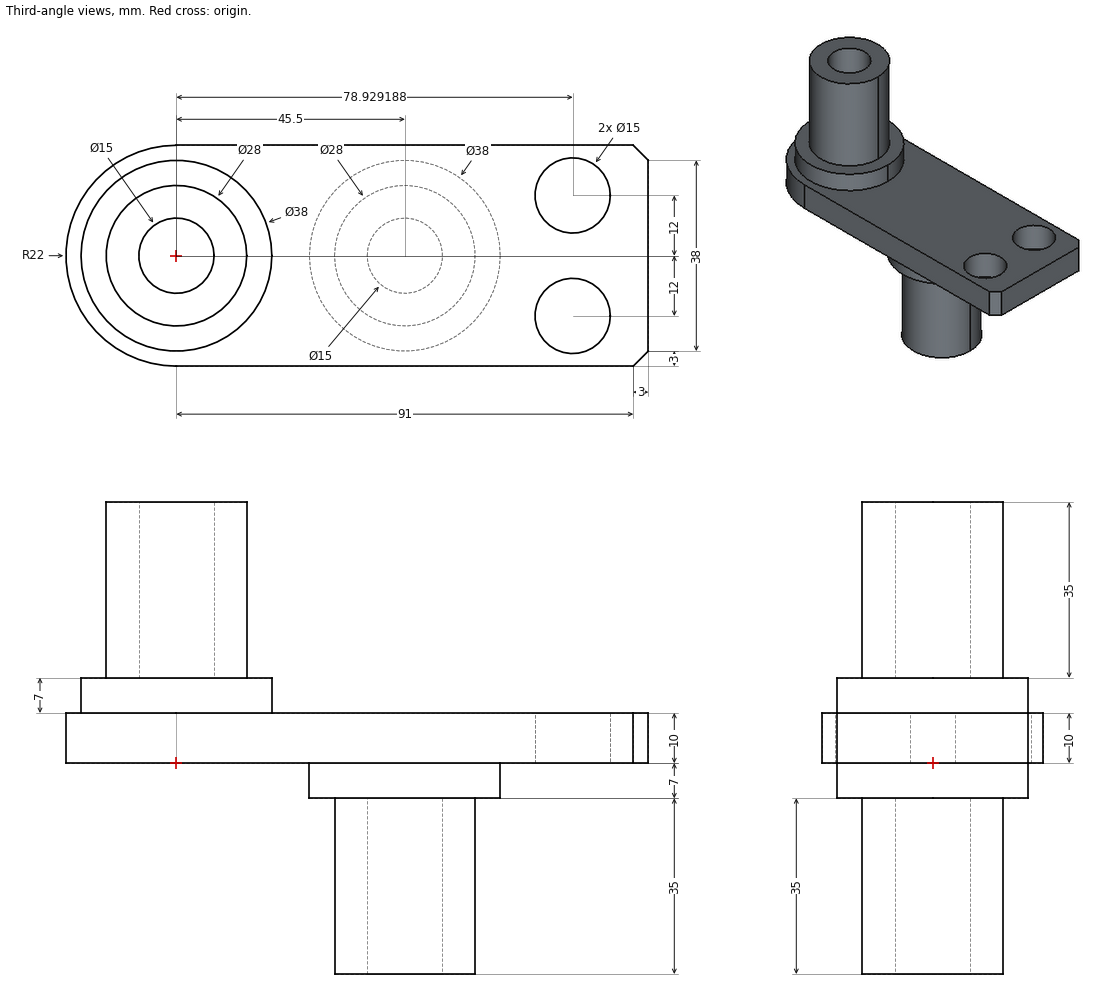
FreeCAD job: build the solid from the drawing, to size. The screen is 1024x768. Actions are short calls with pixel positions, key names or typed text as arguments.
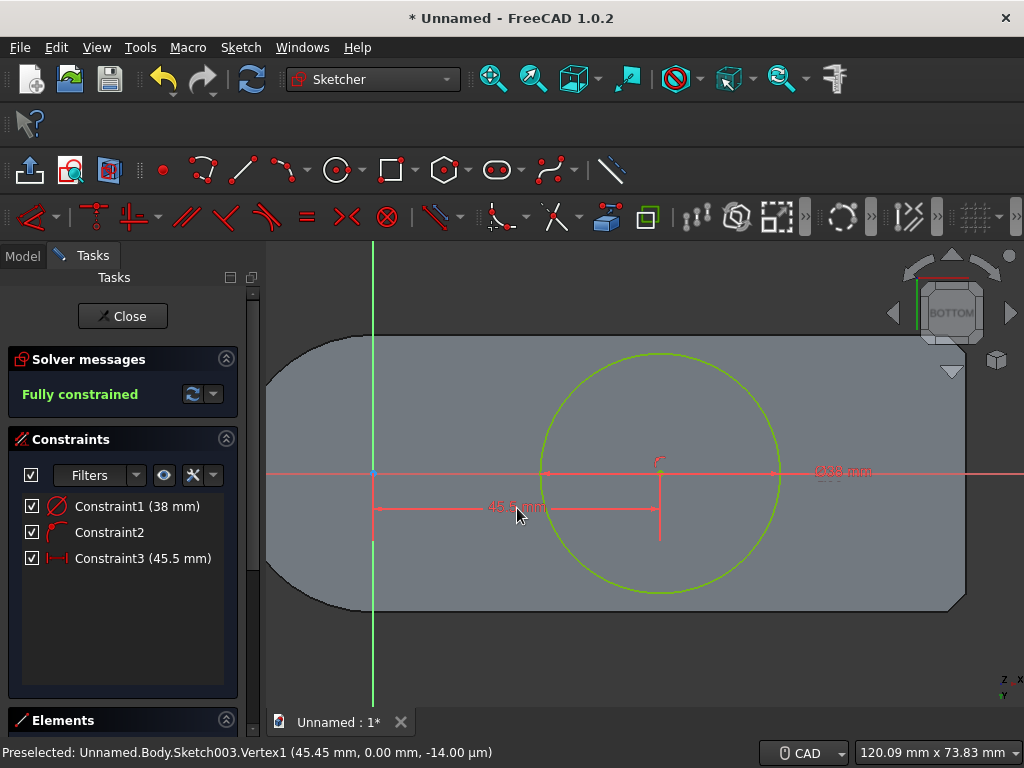
click(123, 316)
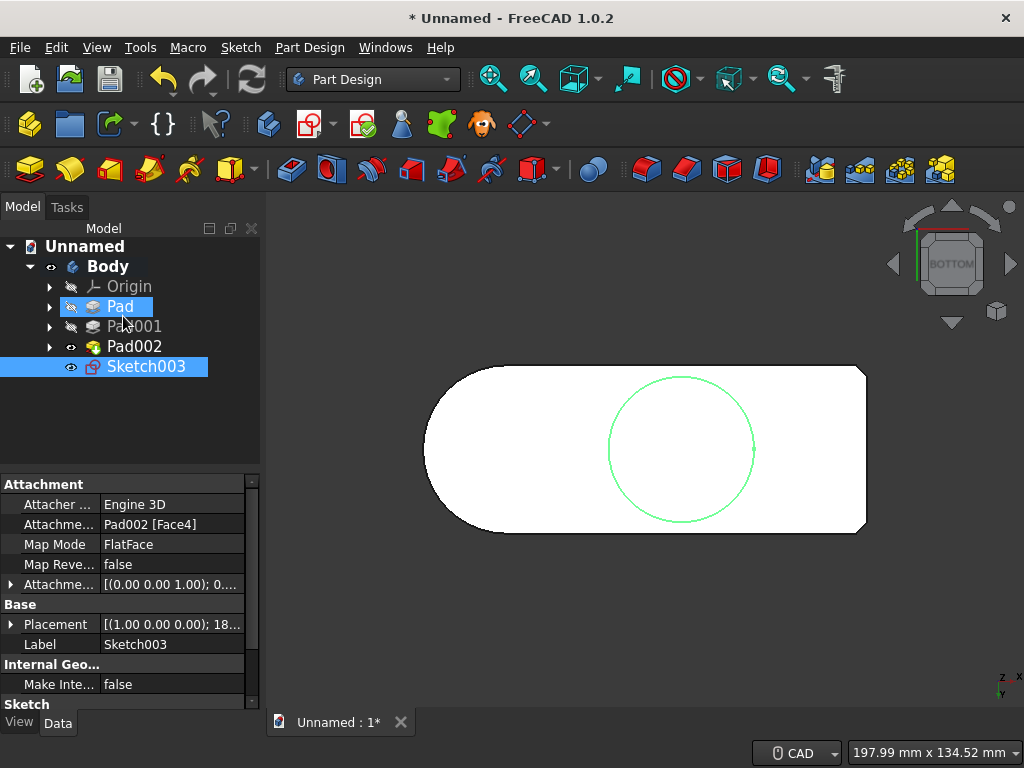
click(30, 170)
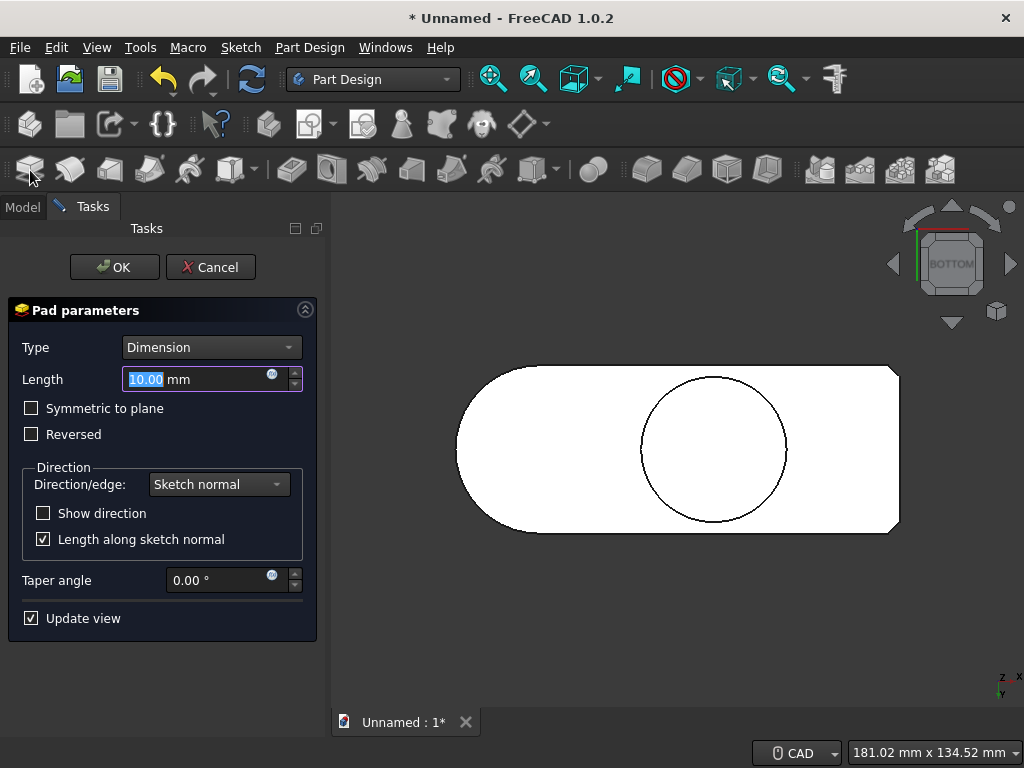
text(7)
key(Tab)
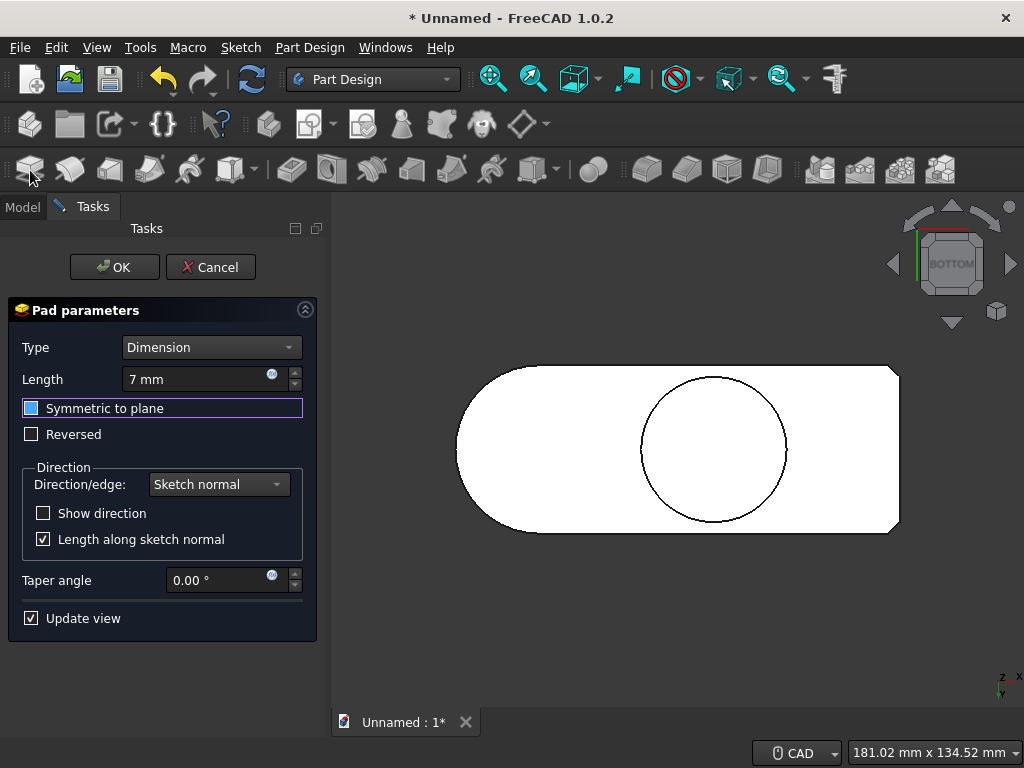
click(115, 267)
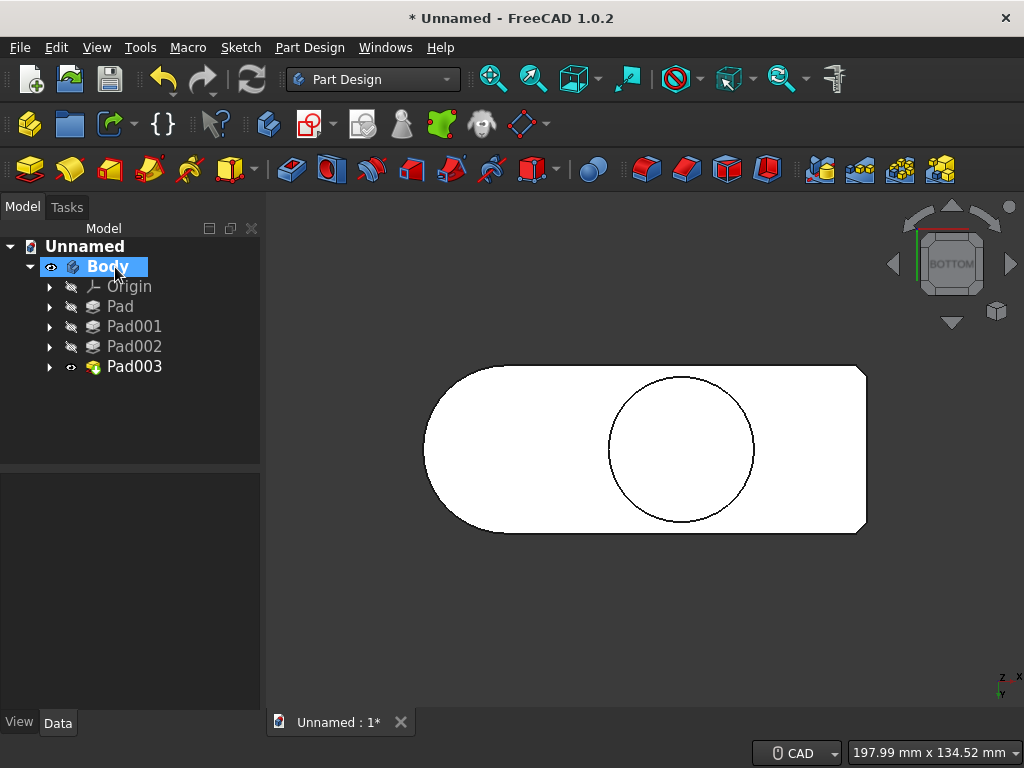
click(681, 449)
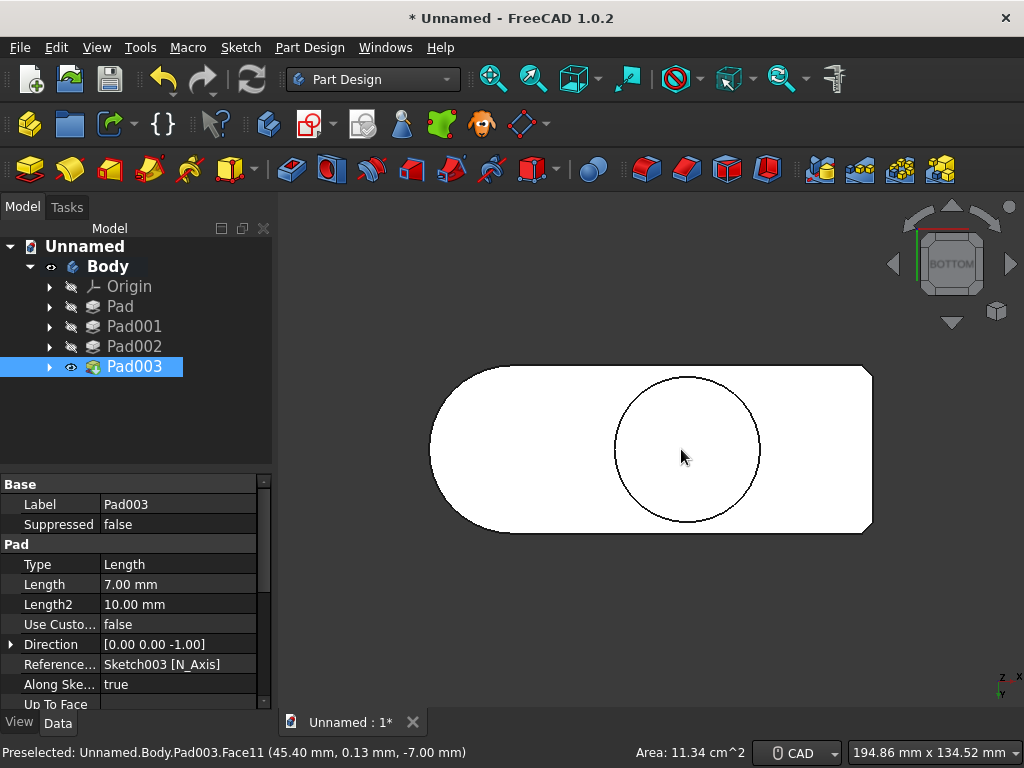
click(310, 124)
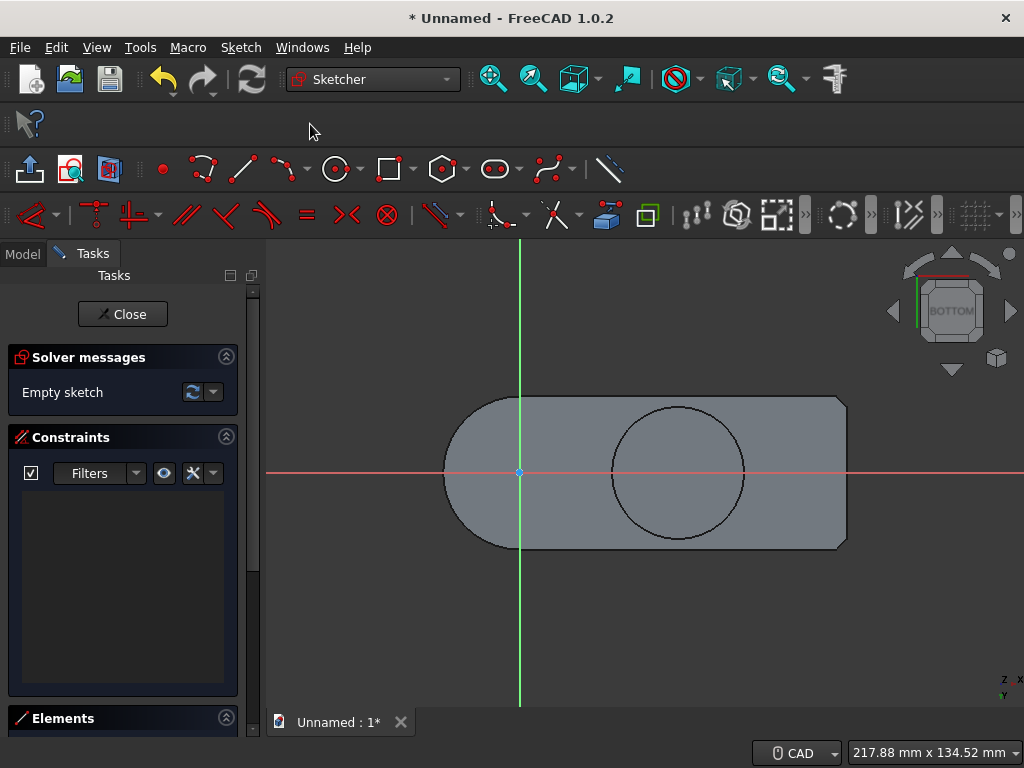
scroll(680, 473, up, 3)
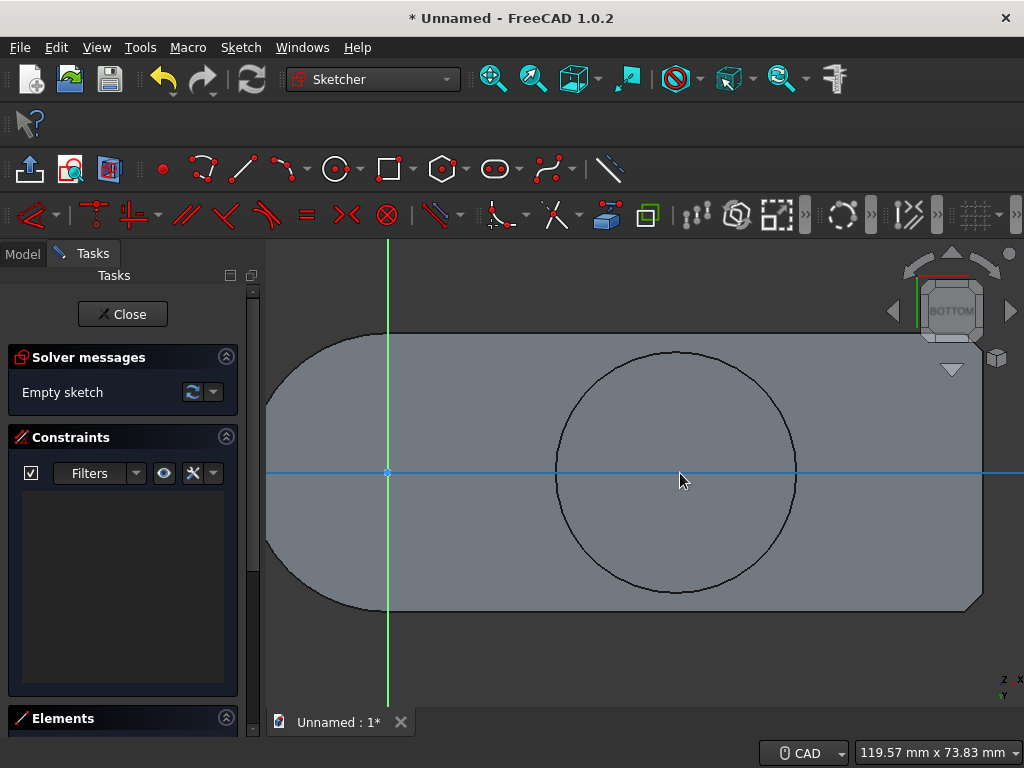
click(336, 170)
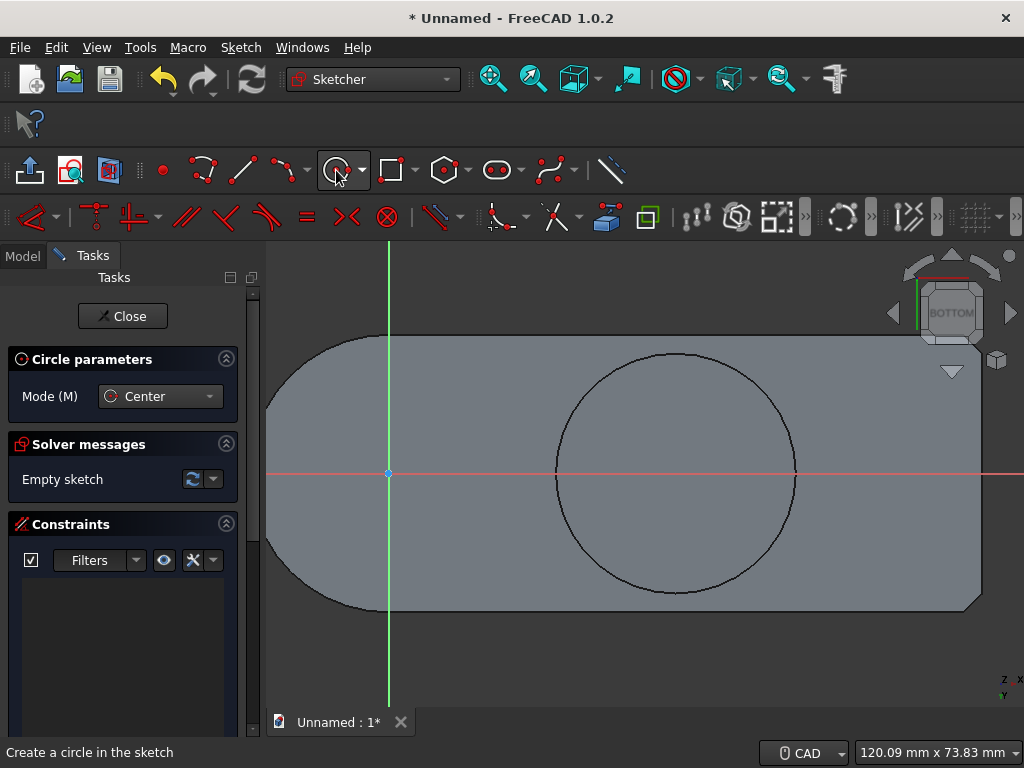
click(676, 474)
move(738, 411)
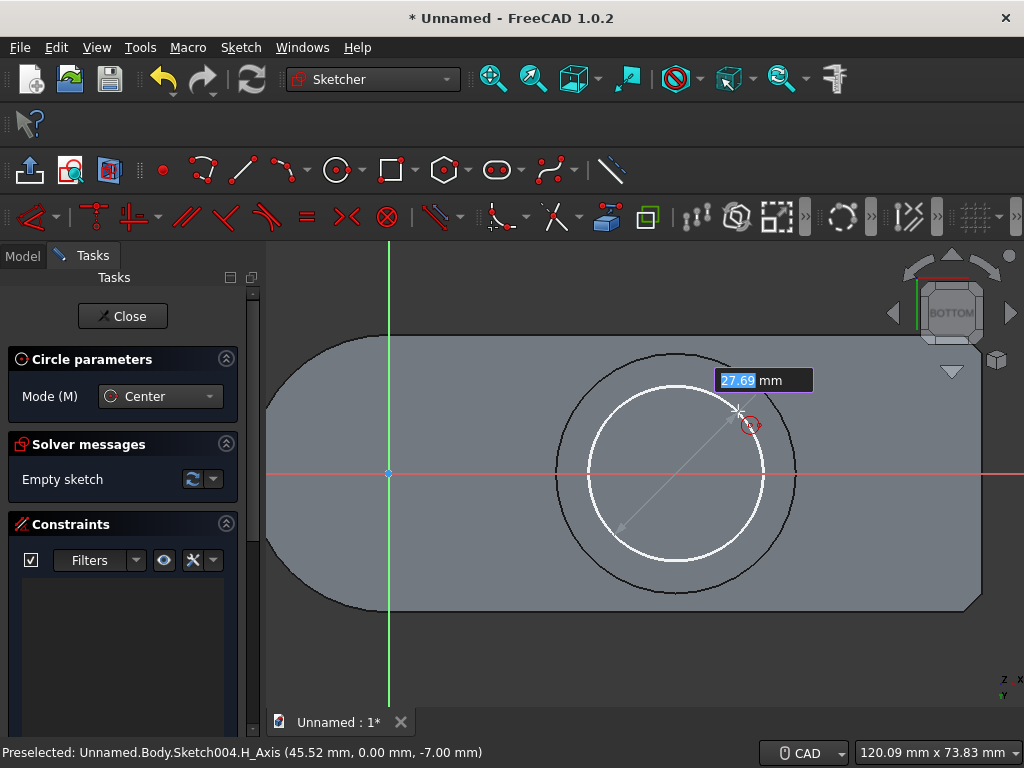
text(28)
key(Return)
key(Escape)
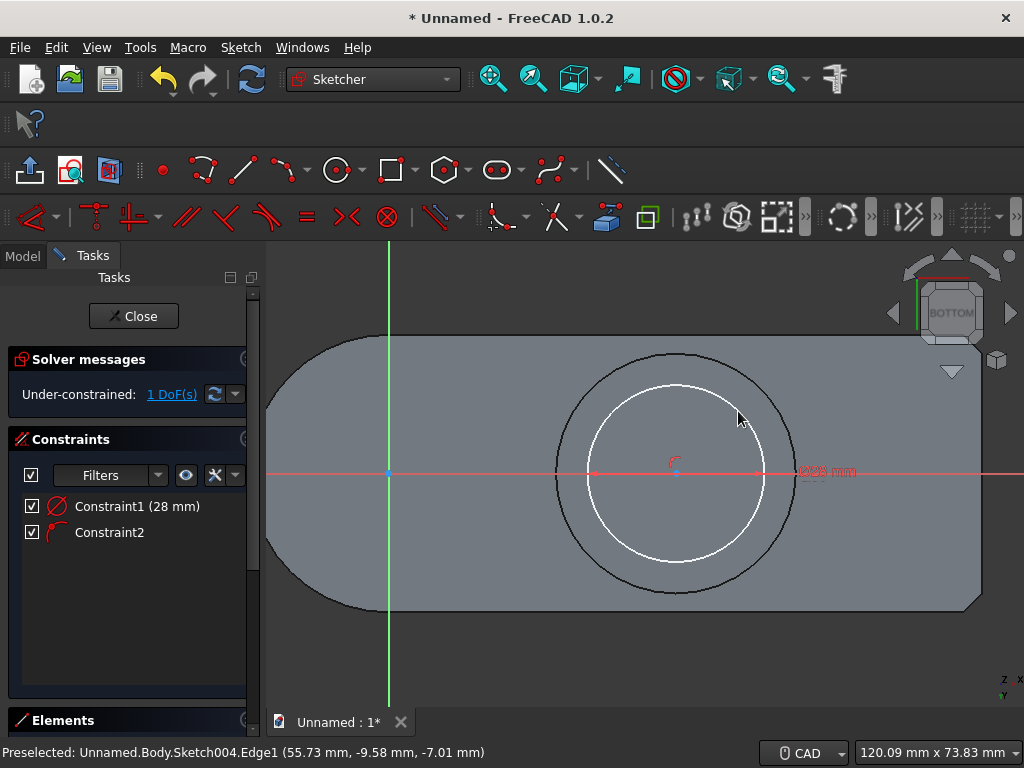
click(32, 218)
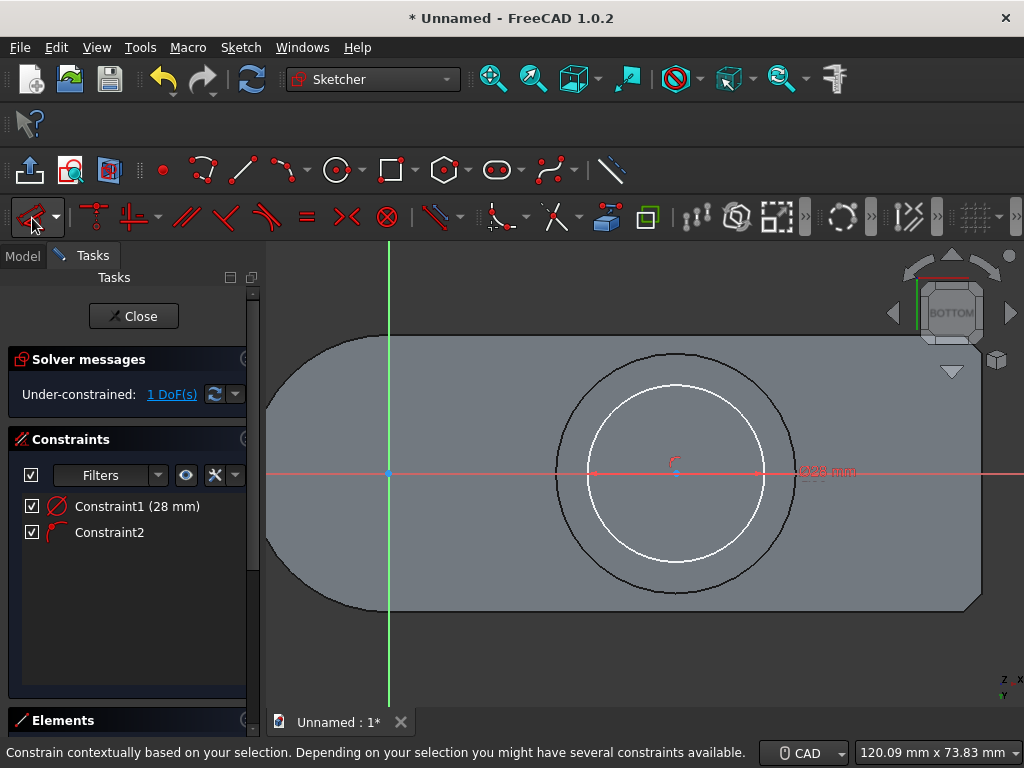
click(676, 474)
click(532, 508)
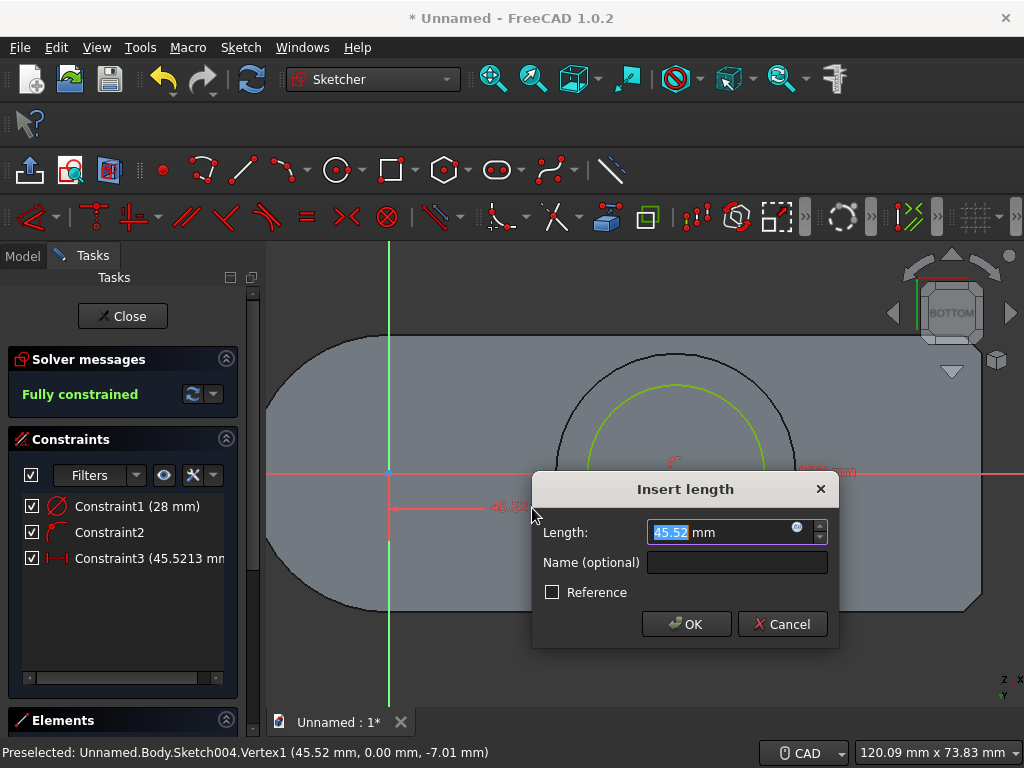
text(45.5)
key(Return)
key(Escape)